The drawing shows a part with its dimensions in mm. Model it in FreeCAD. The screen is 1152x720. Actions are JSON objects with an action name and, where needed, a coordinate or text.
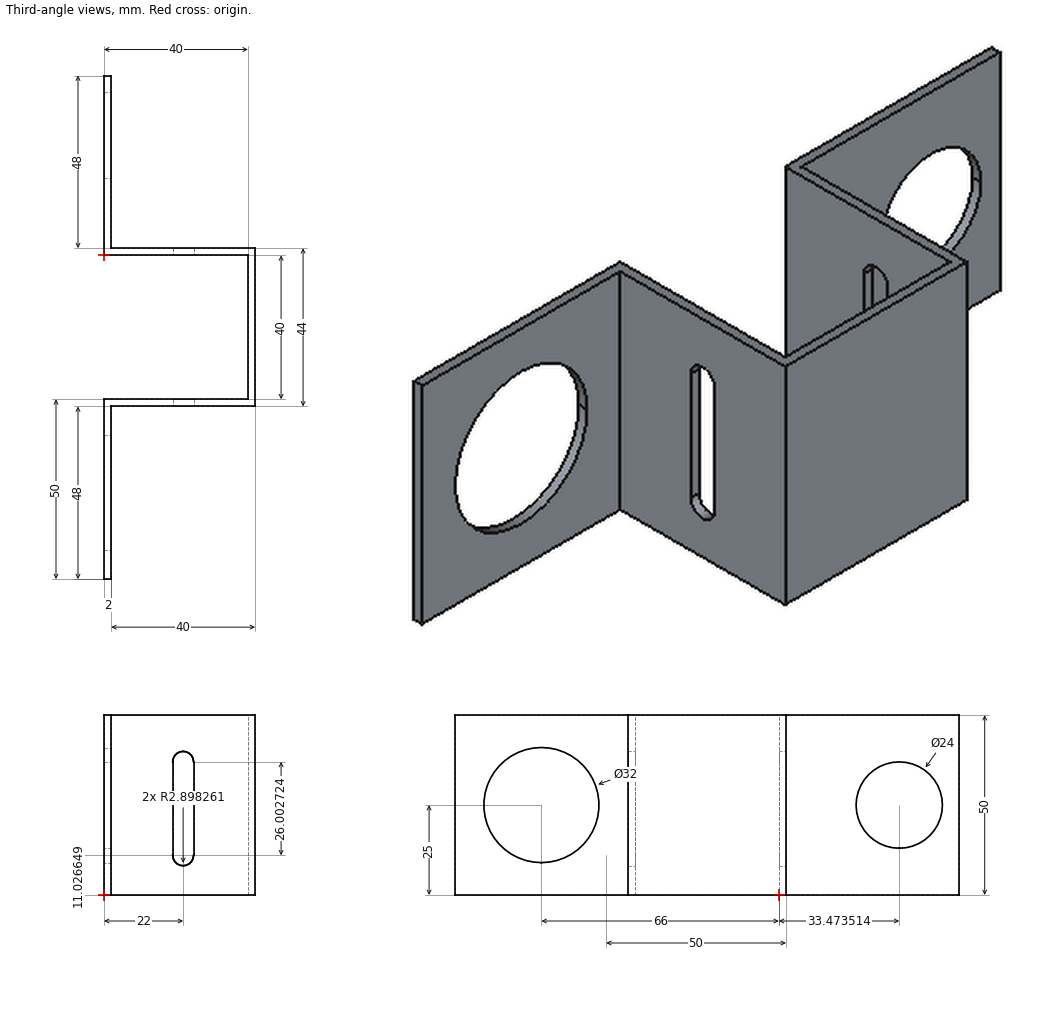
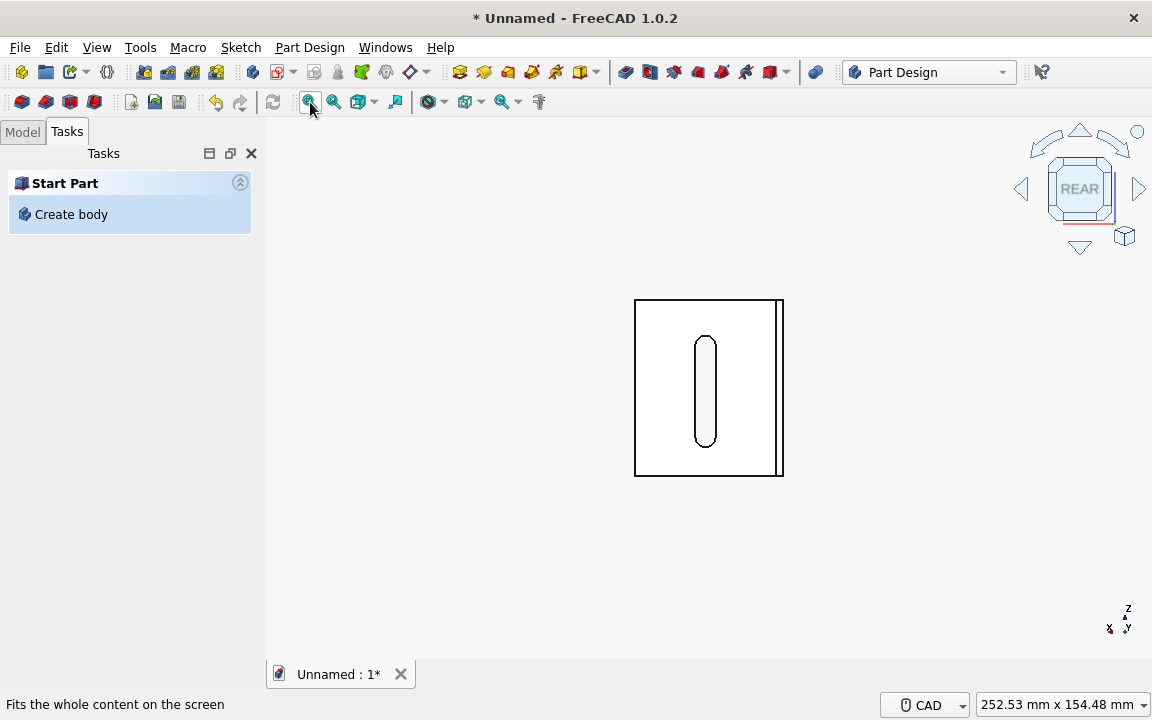
{"action": "key", "text": "0"}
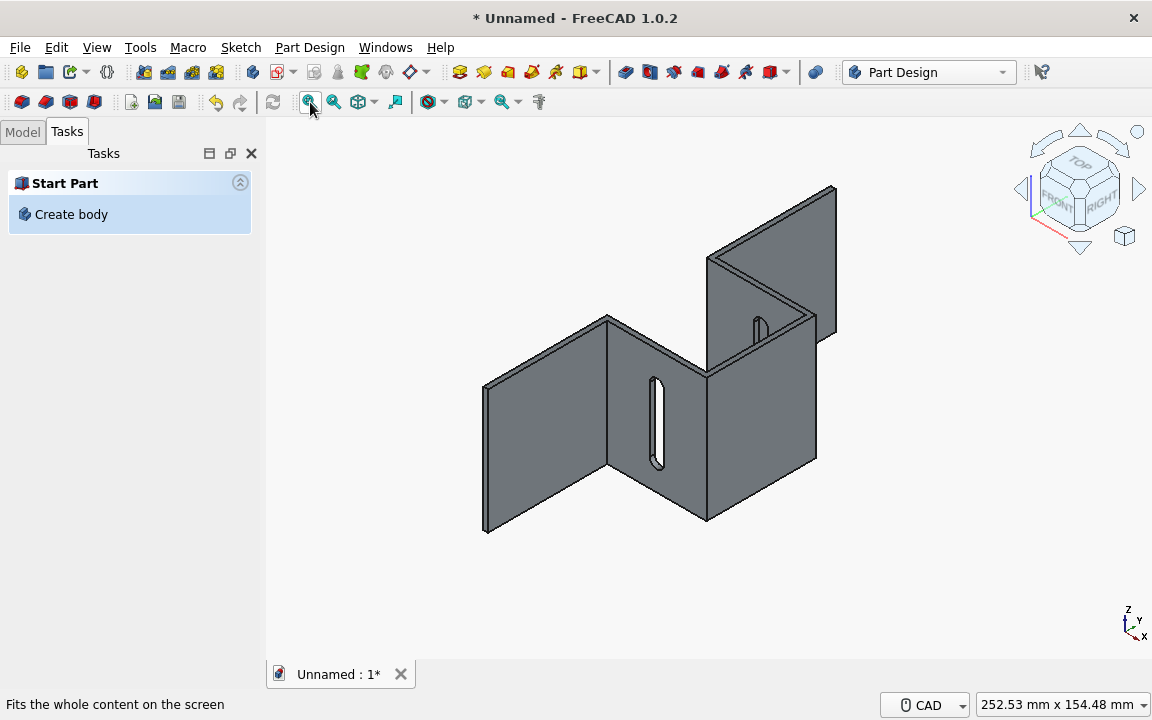
{"action": "left_click", "coordinate": [776, 273]}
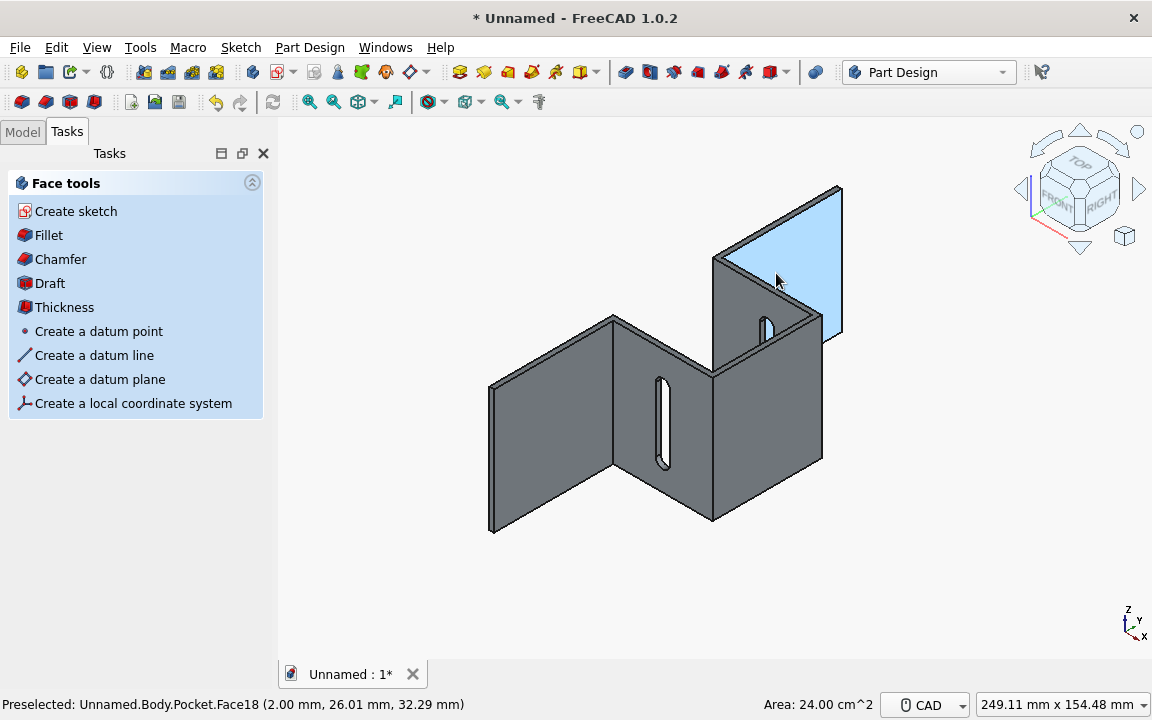
{"action": "left_click", "coordinate": [278, 72]}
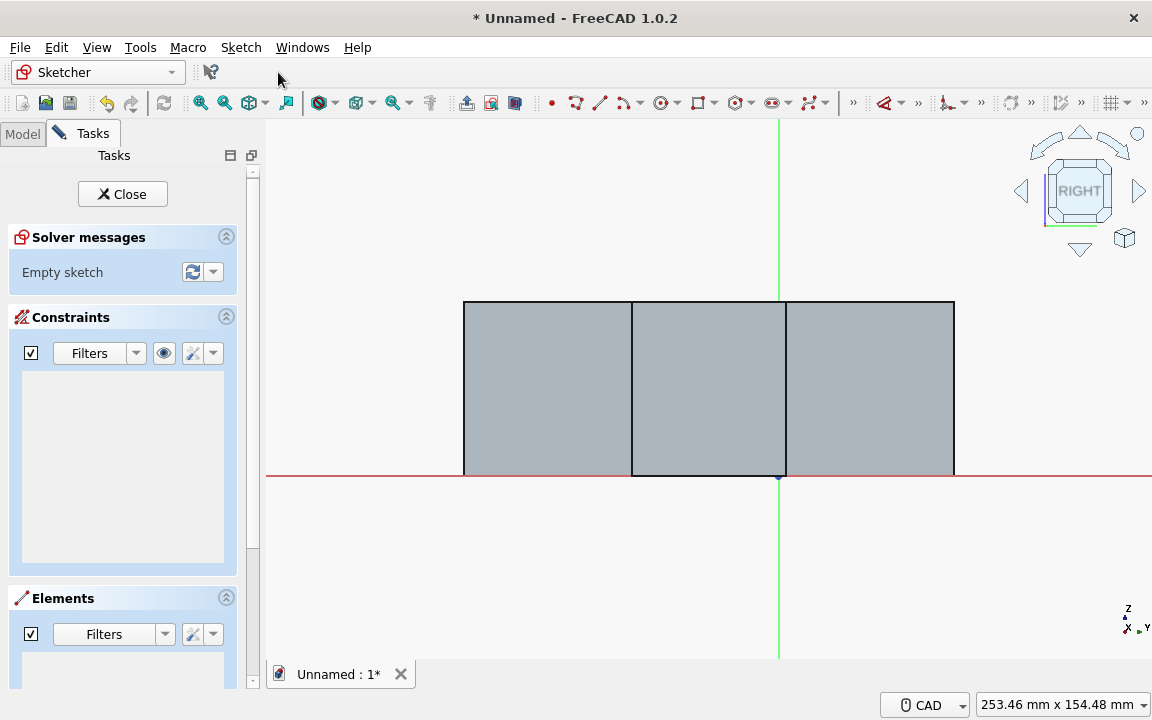
{"action": "scroll", "coordinate": [508, 389], "scroll_direction": "up", "scroll_amount": 6}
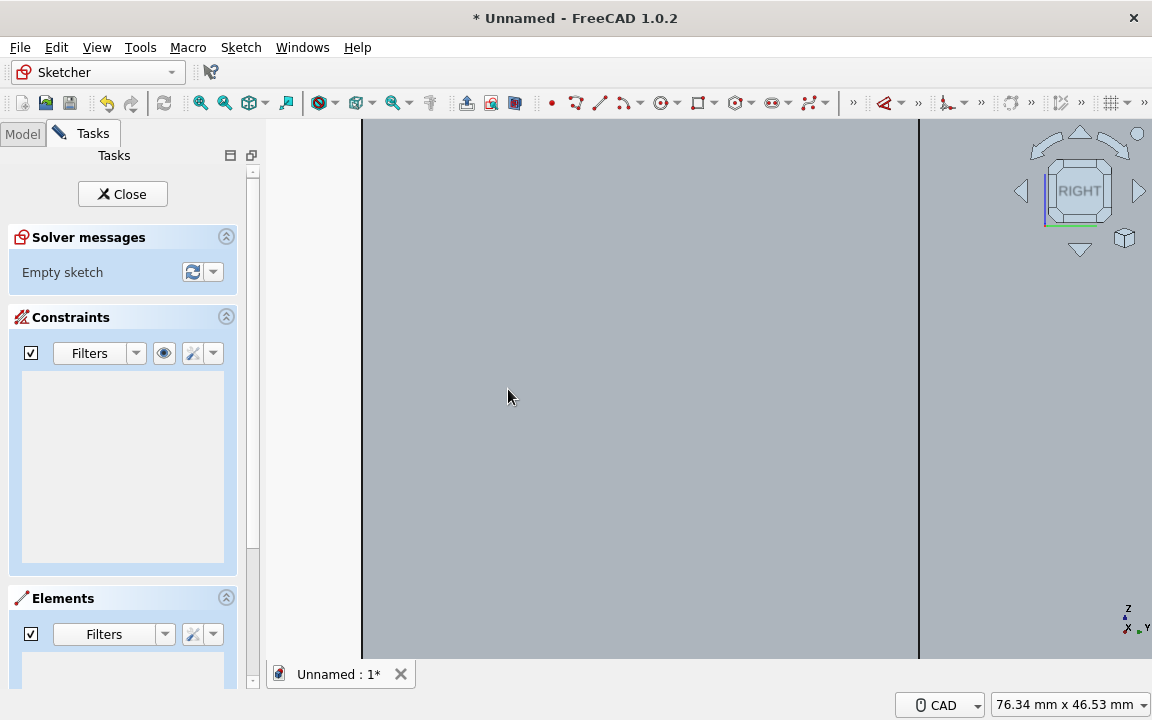
{"action": "left_click", "coordinate": [662, 104]}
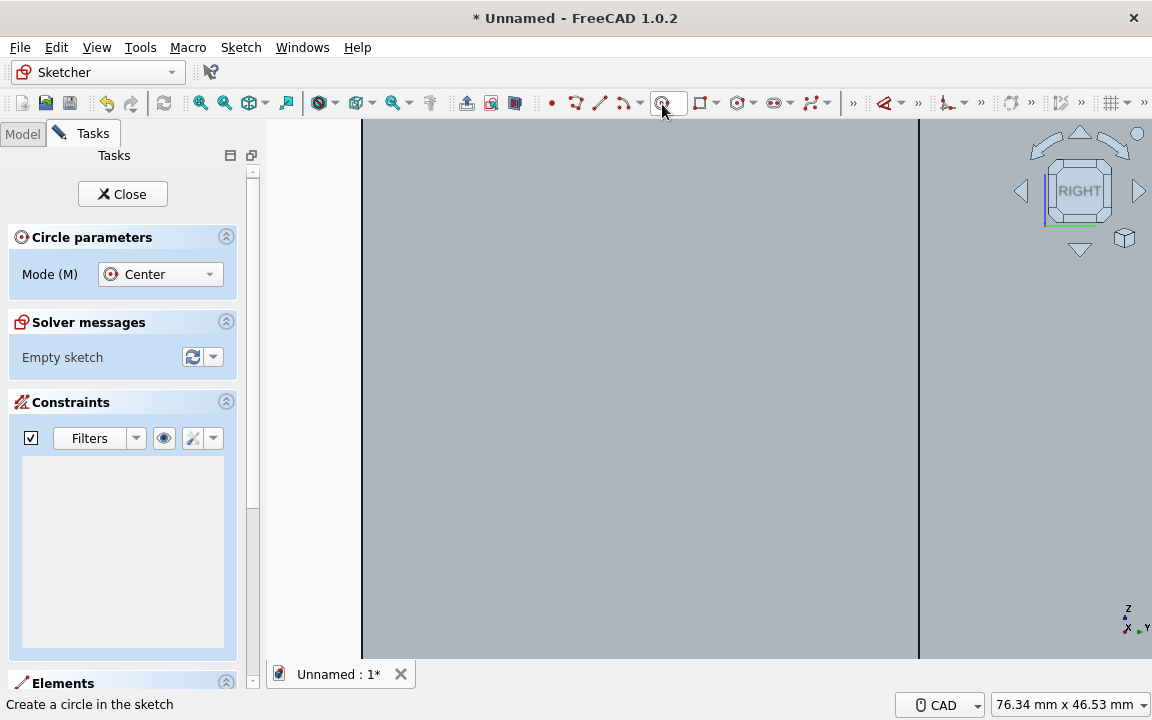
{"action": "left_click", "coordinate": [641, 388]}
{"action": "mouse_move", "coordinate": [772, 257]}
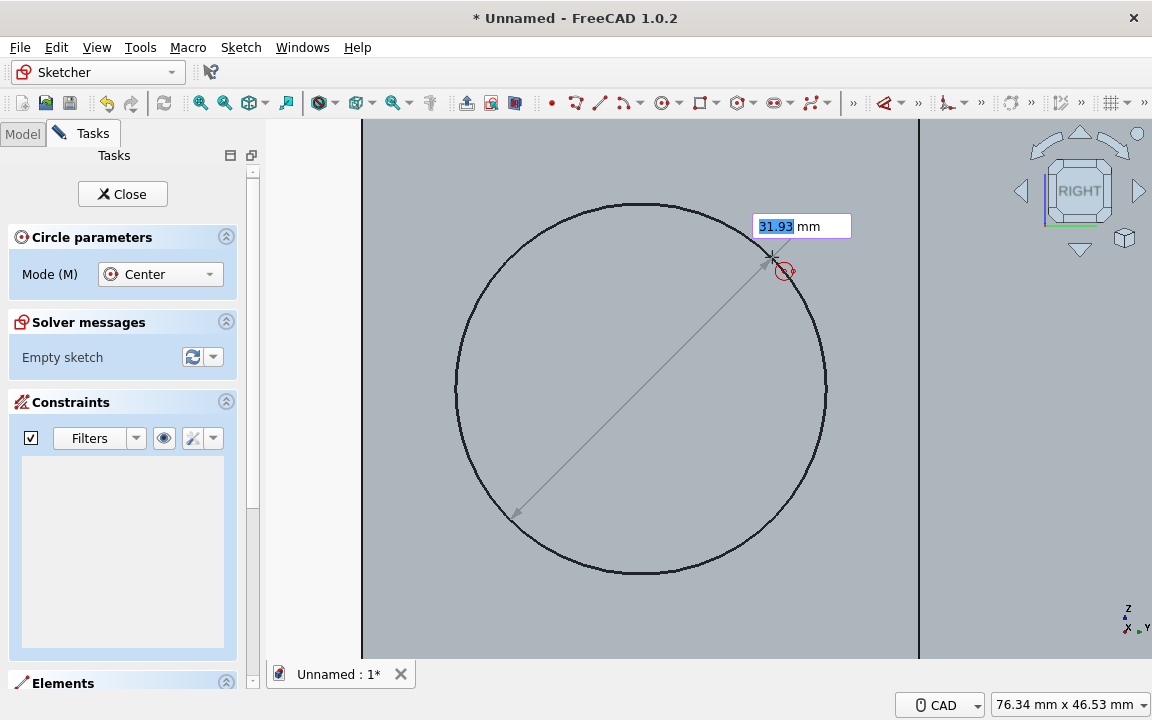
{"action": "type", "text": "32"}
{"action": "key", "text": "Return"}
{"action": "key", "text": "Escape"}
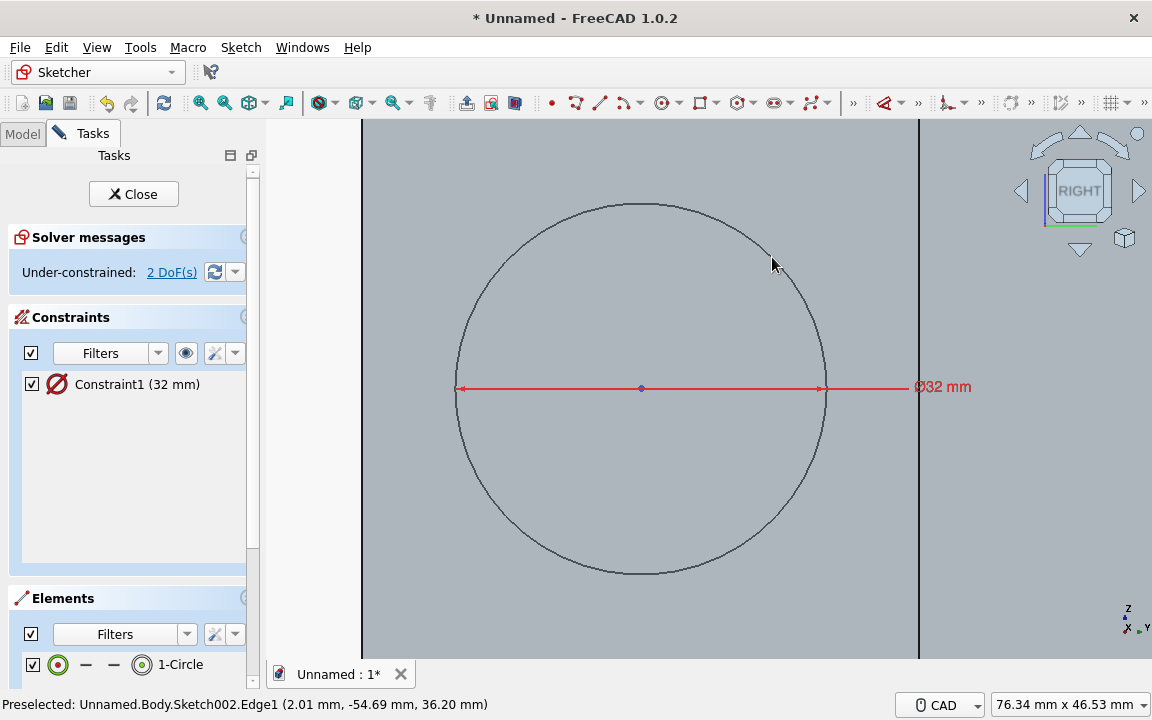
{"action": "key", "text": "d"}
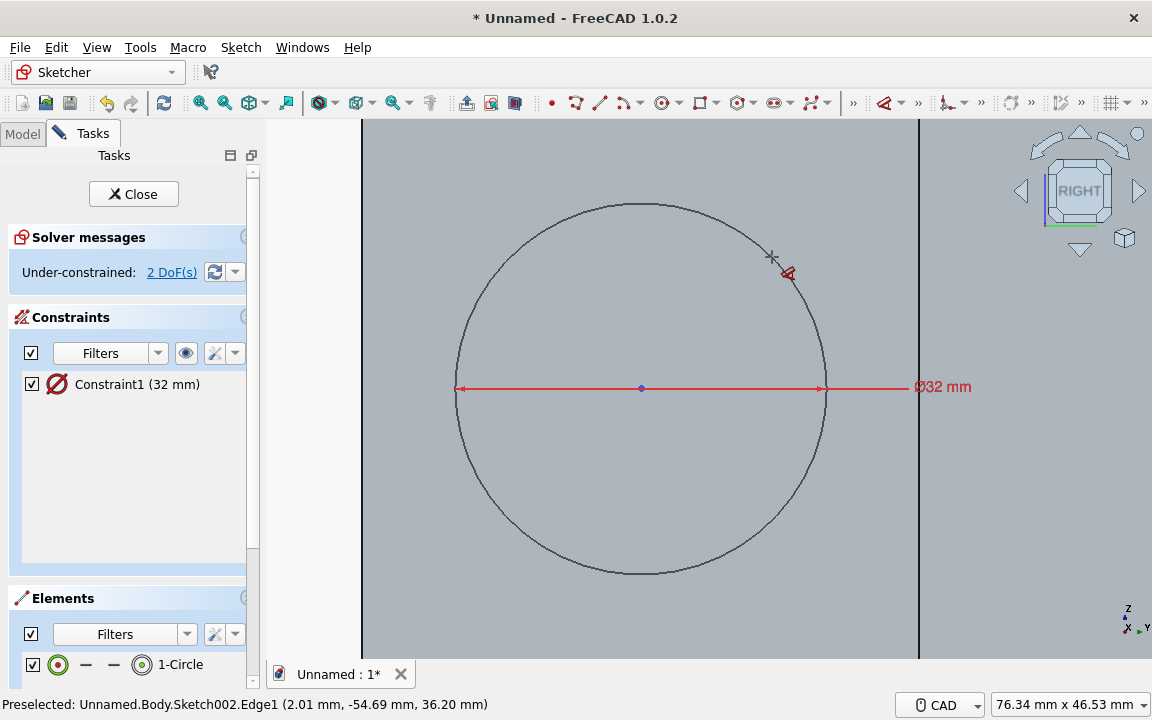
{"action": "left_click", "coordinate": [641, 389]}
{"action": "left_click", "coordinate": [734, 355]}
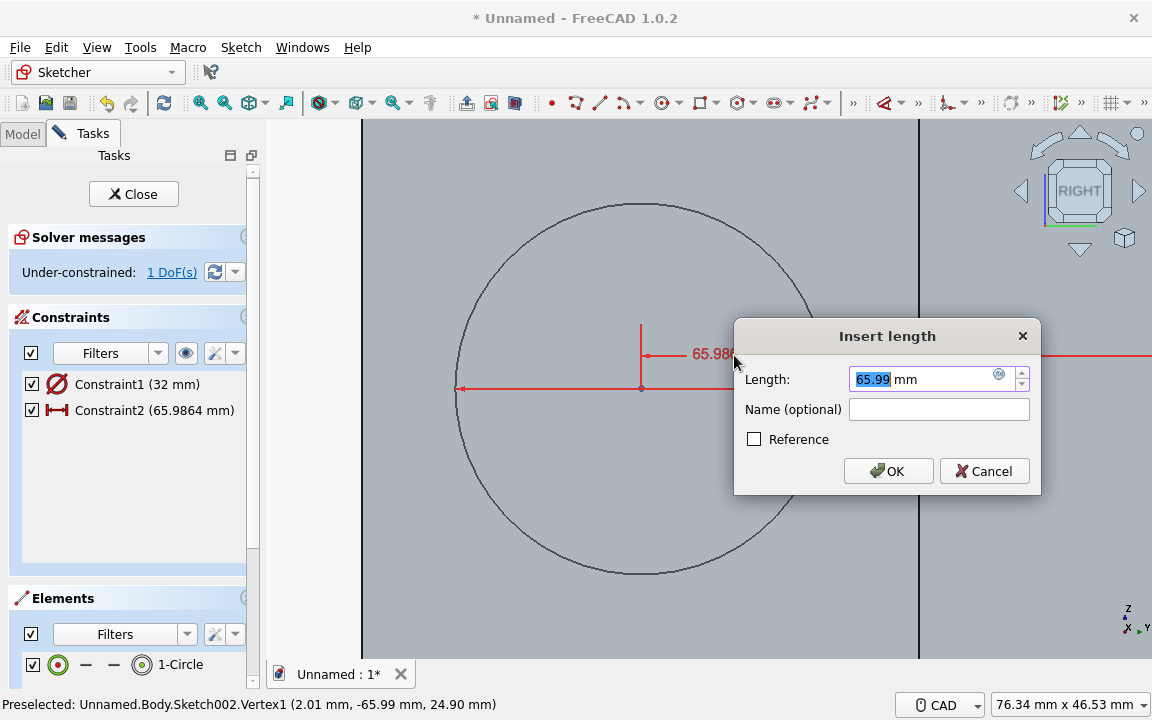
{"action": "type", "text": "66"}
{"action": "key", "text": "Return"}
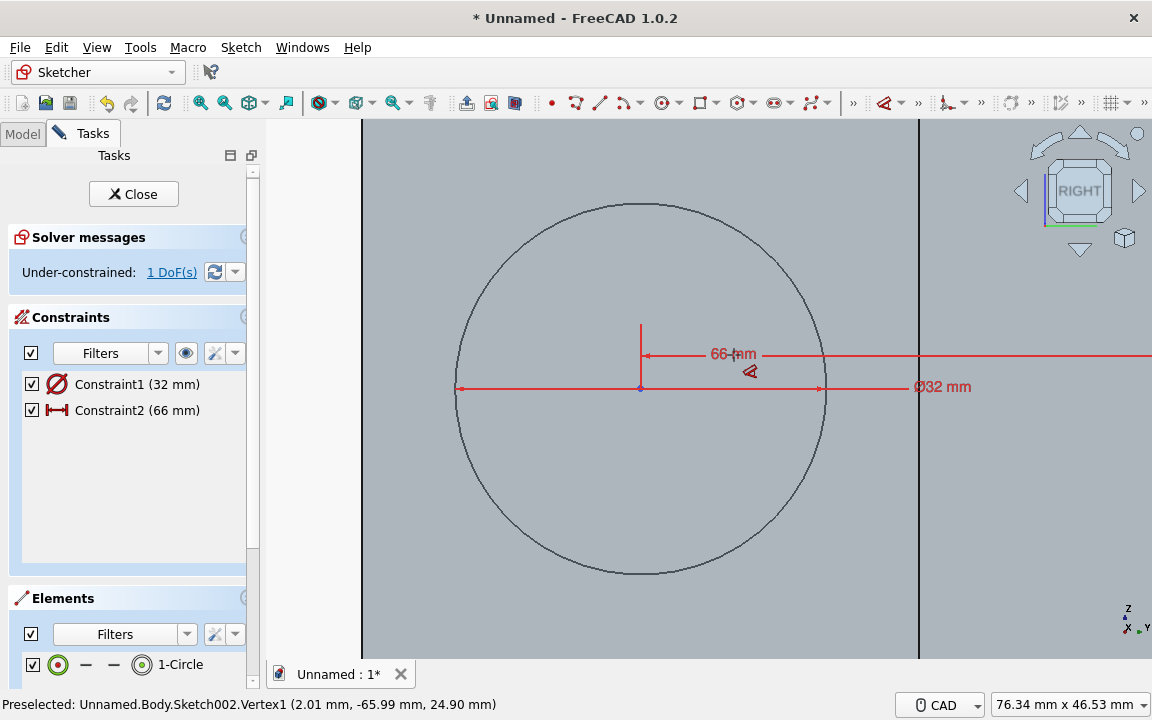
{"action": "left_click", "coordinate": [641, 389]}
{"action": "left_click", "coordinate": [607, 510]}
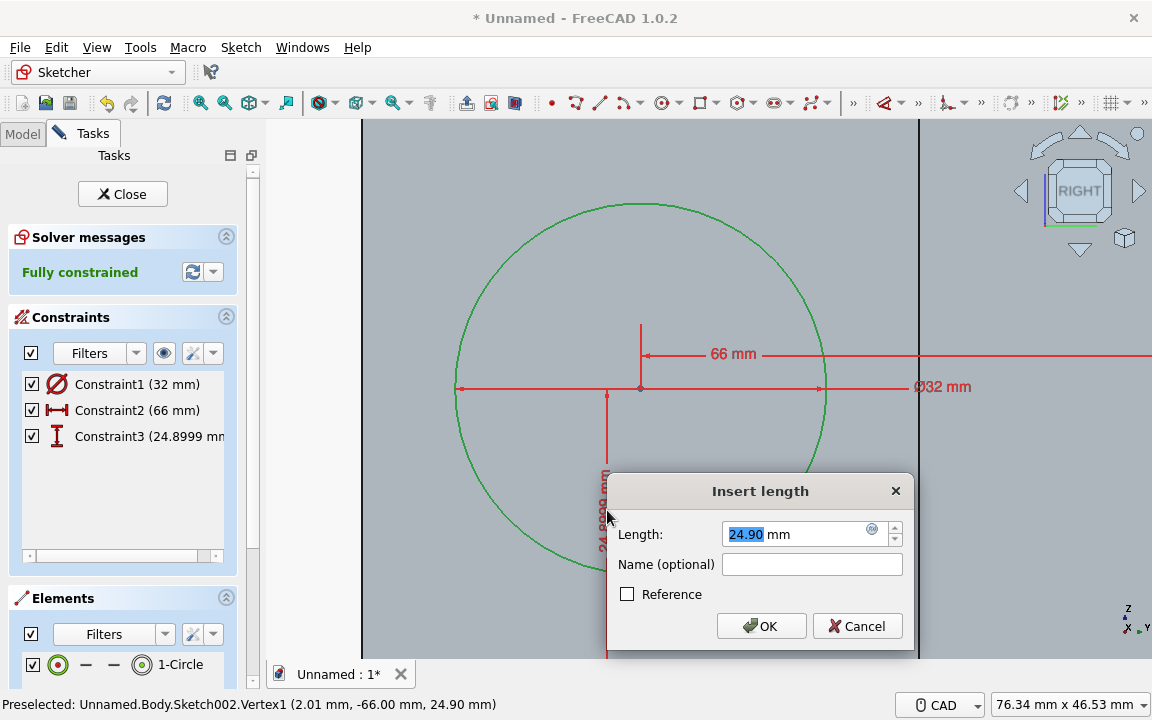
{"action": "type", "text": "25"}
{"action": "key", "text": "Return"}
{"action": "key", "text": "Escape"}